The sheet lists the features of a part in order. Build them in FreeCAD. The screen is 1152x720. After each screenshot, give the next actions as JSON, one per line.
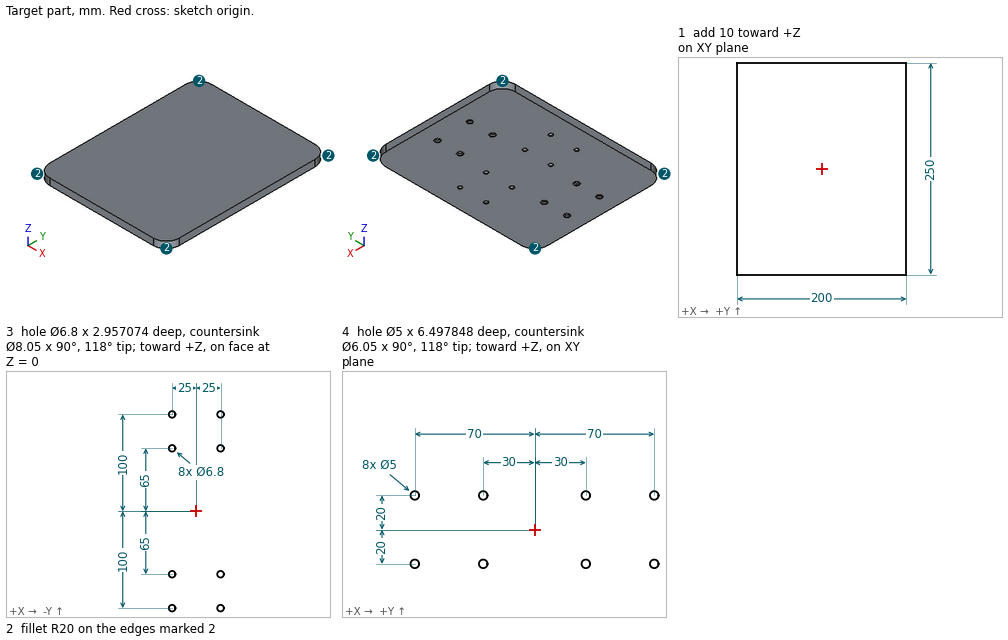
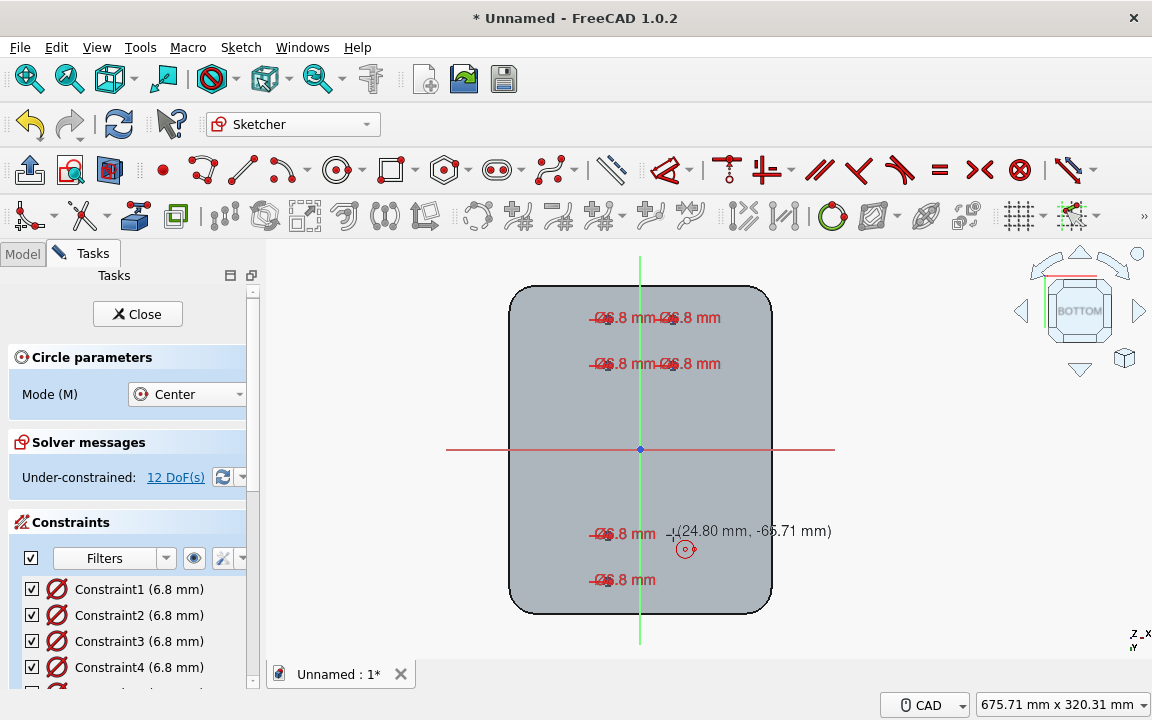
{"action": "left_click", "coordinate": [673, 535]}
{"action": "mouse_move", "coordinate": [676, 532]}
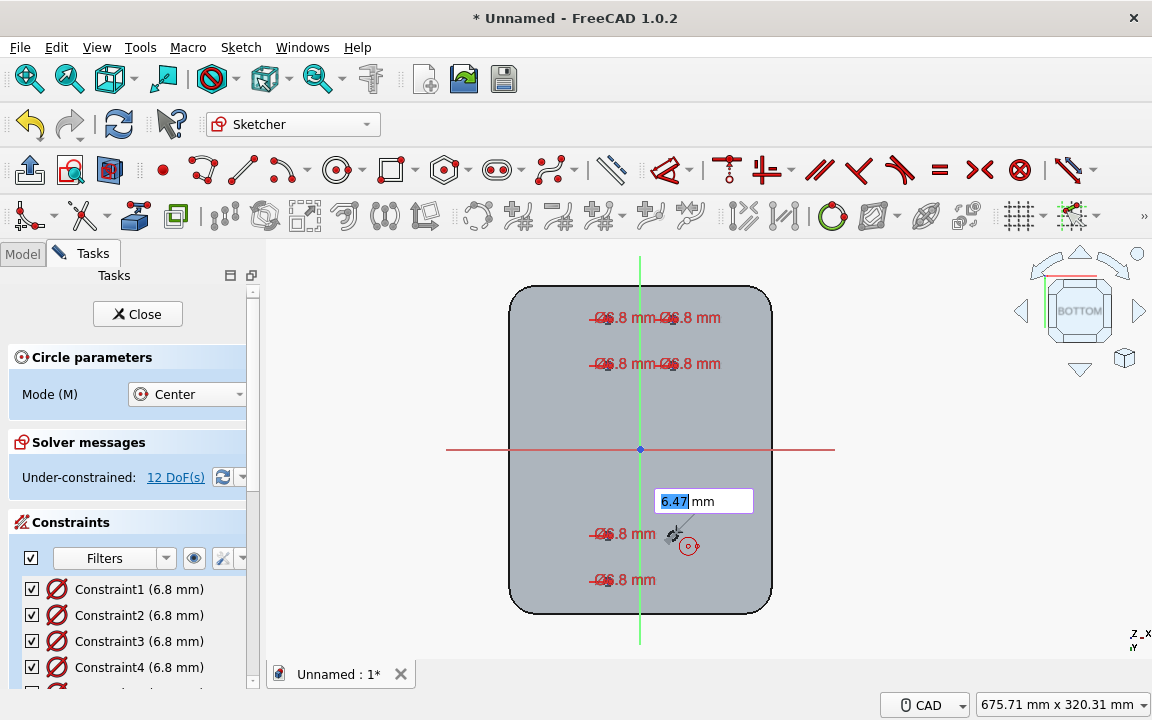
{"action": "type", "text": "6.8"}
{"action": "key", "text": "Return"}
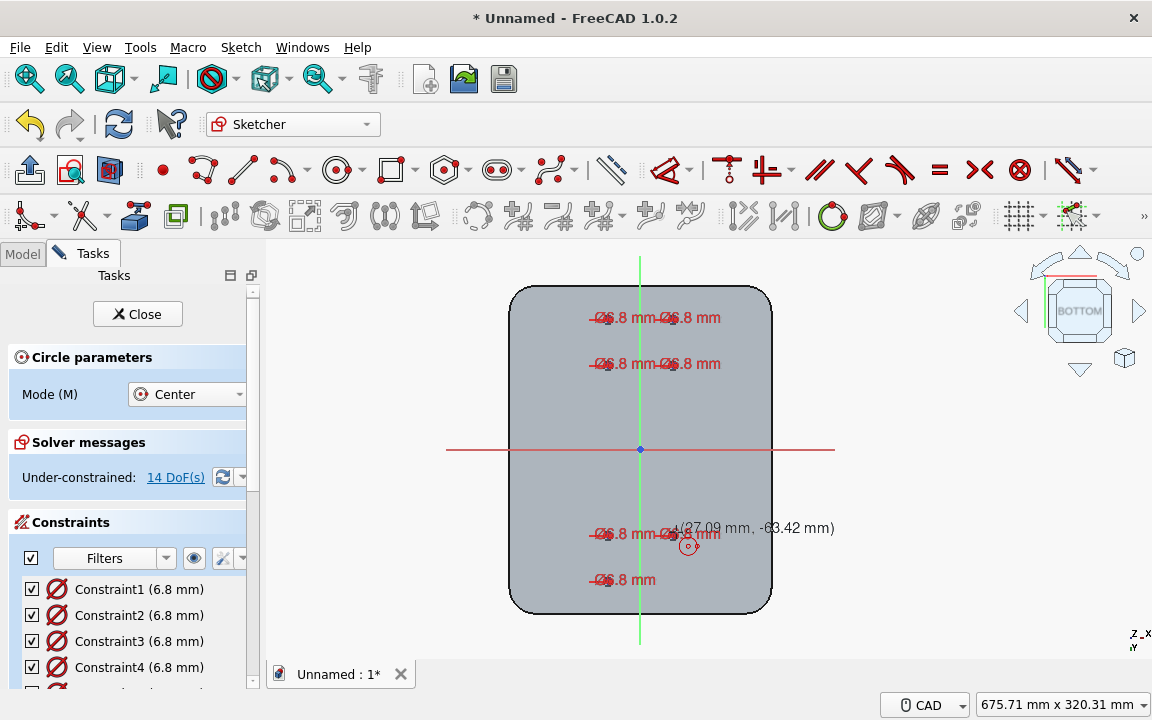
{"action": "scroll", "coordinate": [673, 581], "scroll_direction": "up", "scroll_amount": 9}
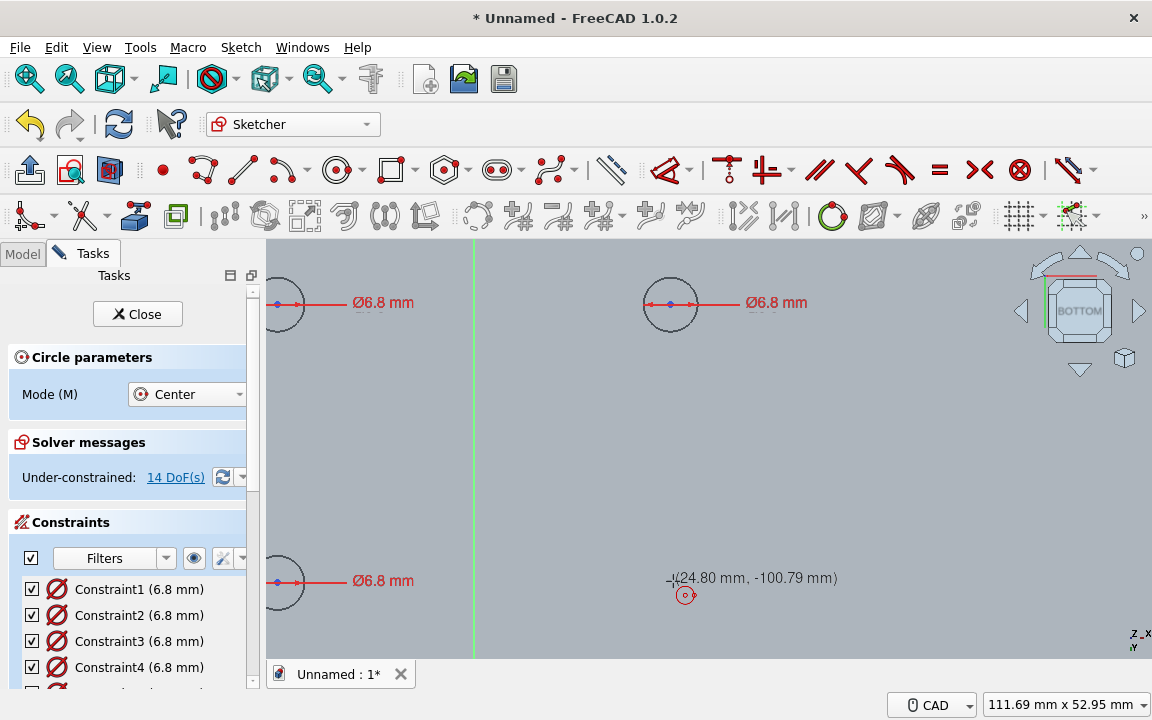
{"action": "scroll", "coordinate": [673, 581], "scroll_direction": "down", "scroll_amount": 9}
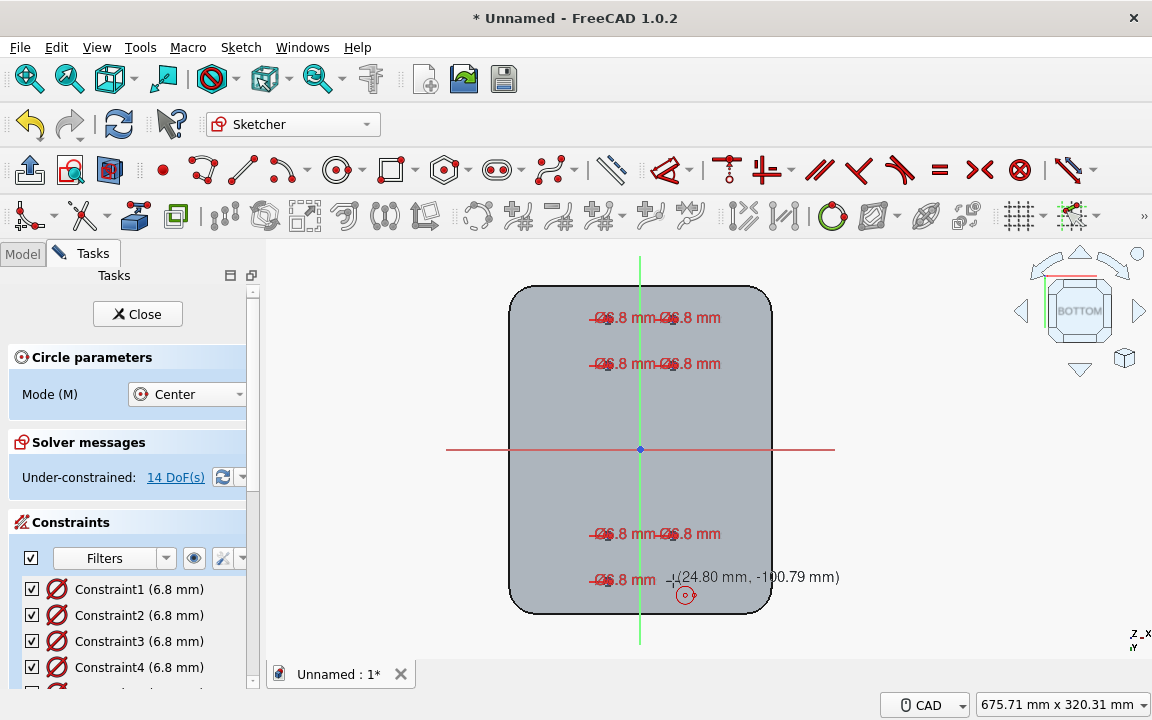
{"action": "left_click", "coordinate": [673, 581]}
{"action": "mouse_move", "coordinate": [676, 578]}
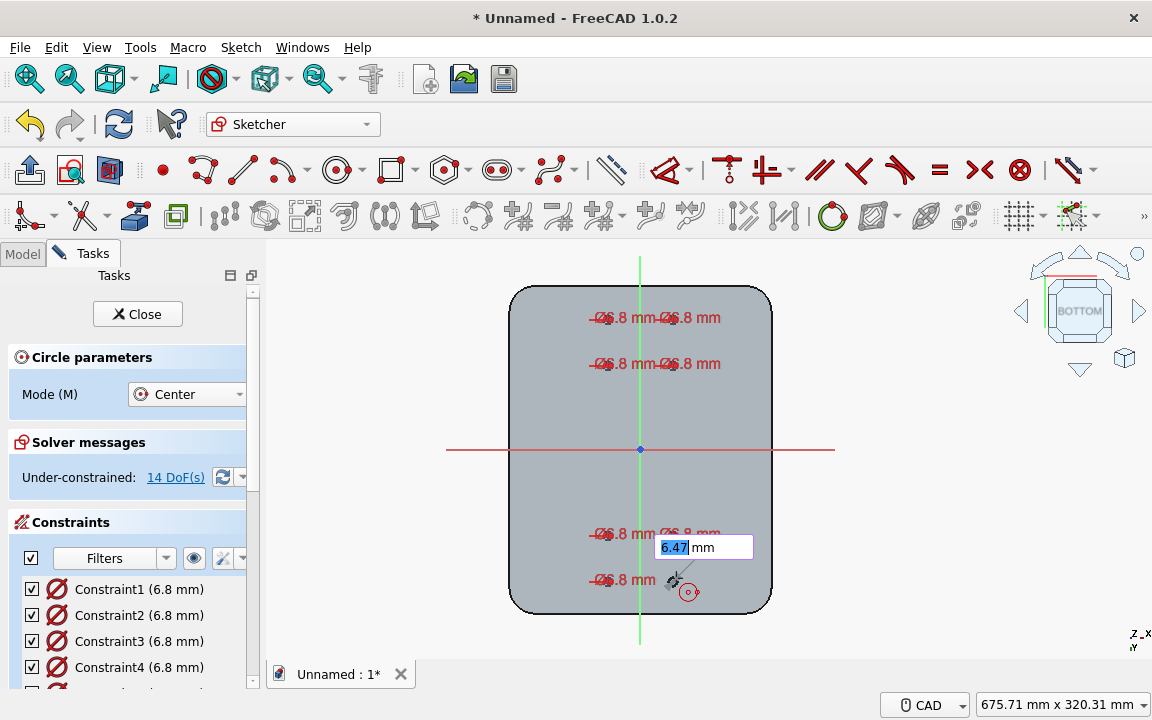
{"action": "type", "text": "6.8"}
{"action": "key", "text": "Return"}
{"action": "key", "text": "Escape"}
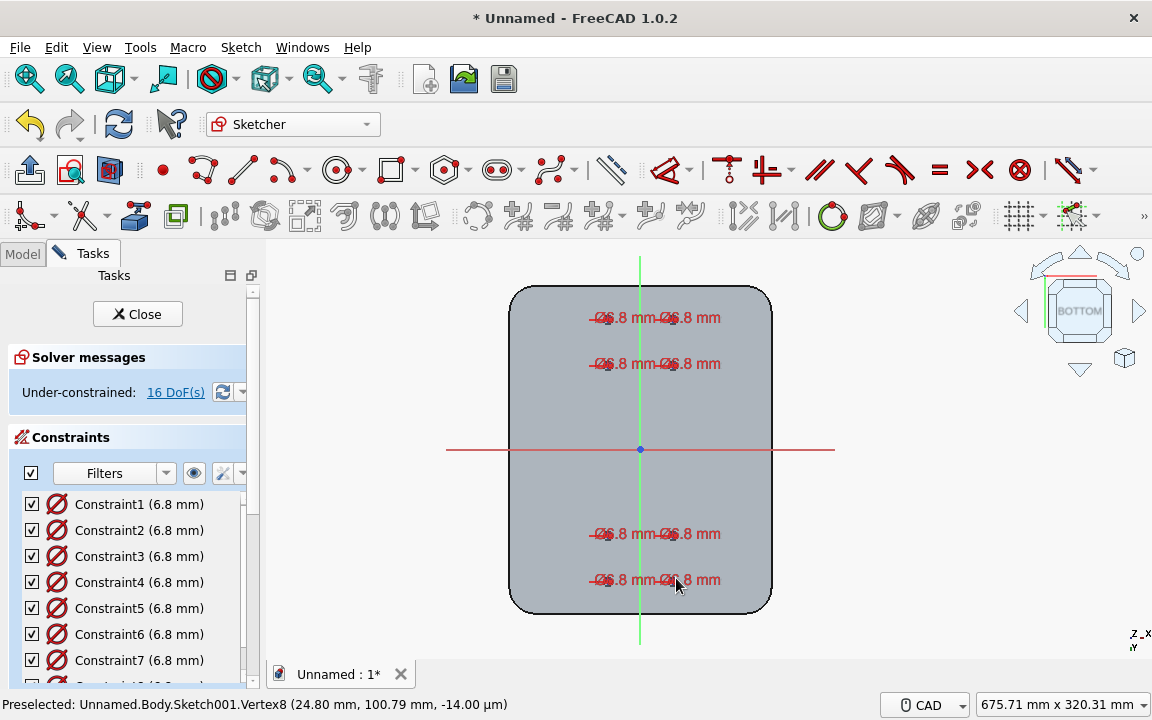
{"action": "left_click", "coordinate": [608, 320]}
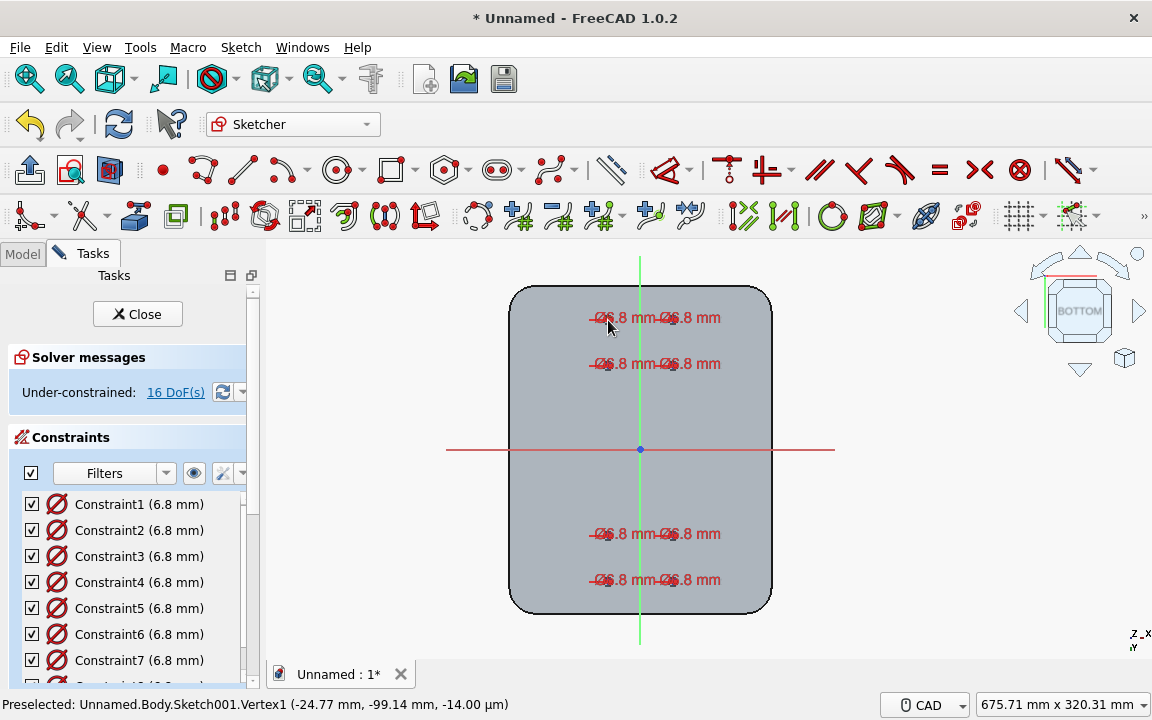
{"action": "left_click", "coordinate": [608, 366]}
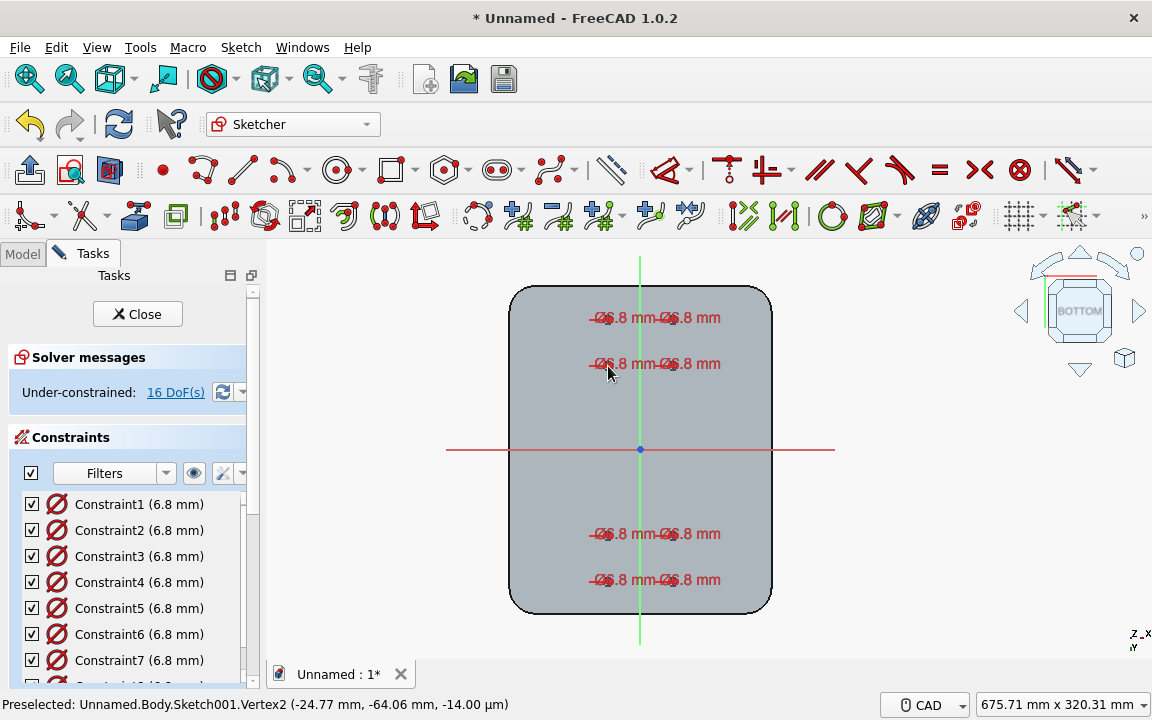
{"action": "left_click", "coordinate": [794, 170]}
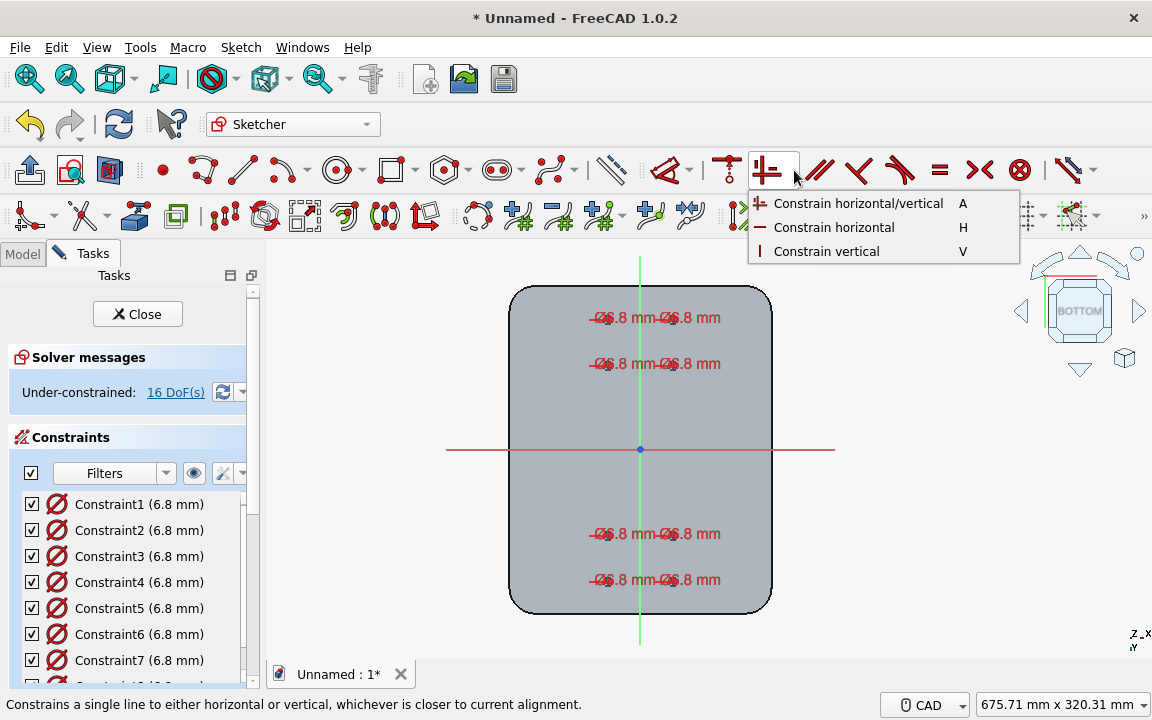
{"action": "left_click", "coordinate": [884, 251]}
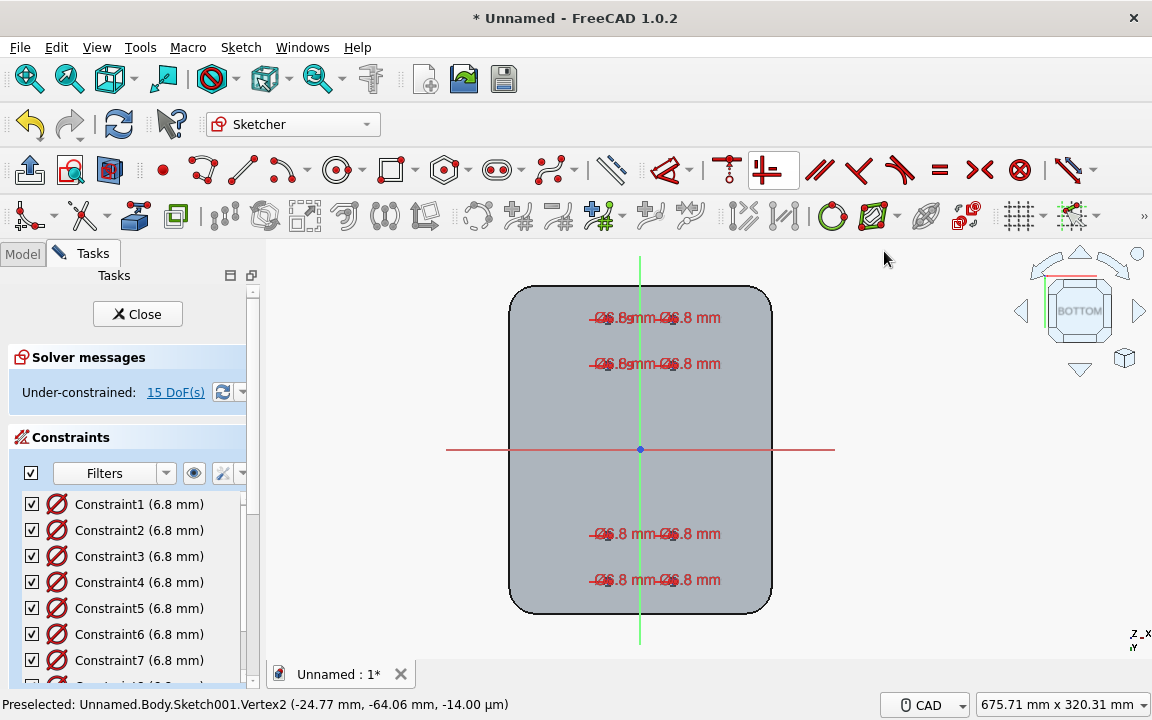
{"action": "left_click", "coordinate": [608, 366]}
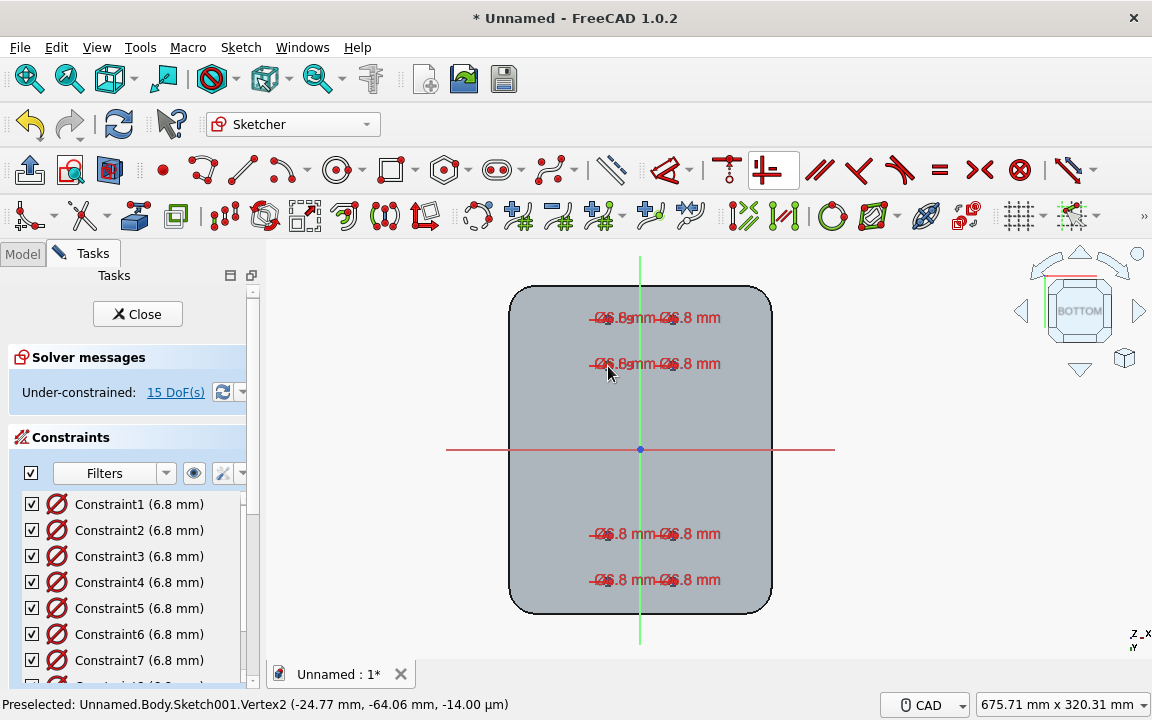
{"action": "left_click", "coordinate": [673, 366]}